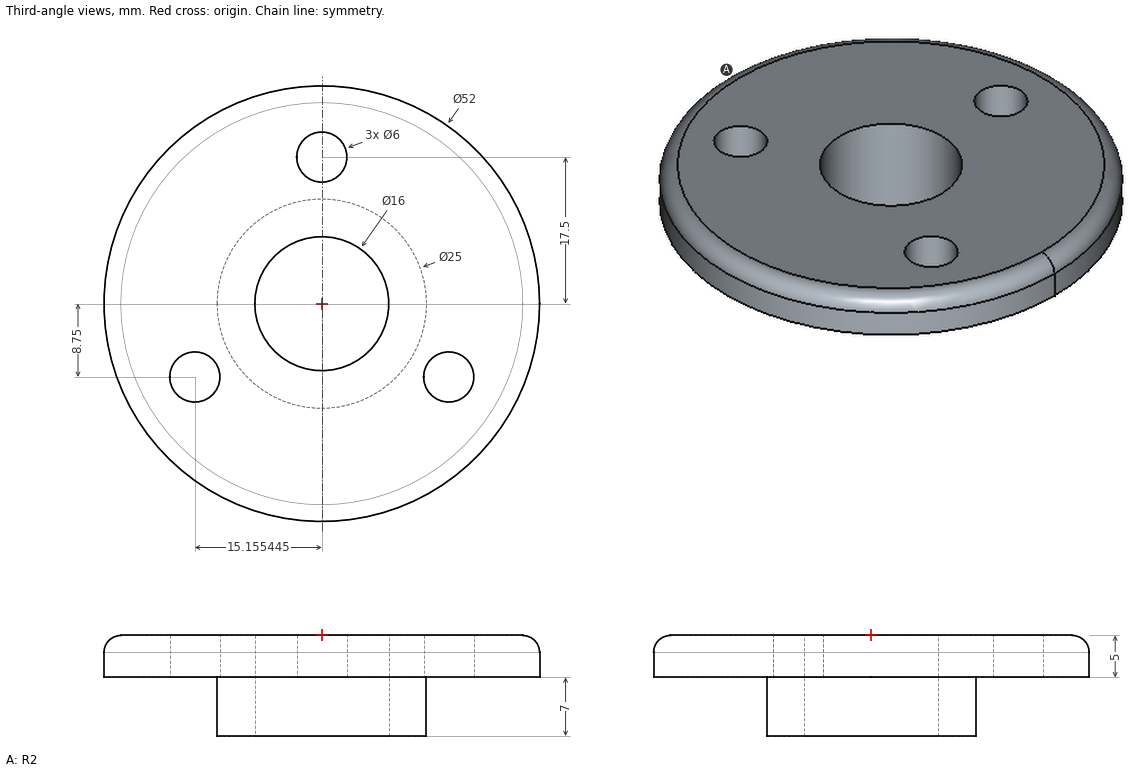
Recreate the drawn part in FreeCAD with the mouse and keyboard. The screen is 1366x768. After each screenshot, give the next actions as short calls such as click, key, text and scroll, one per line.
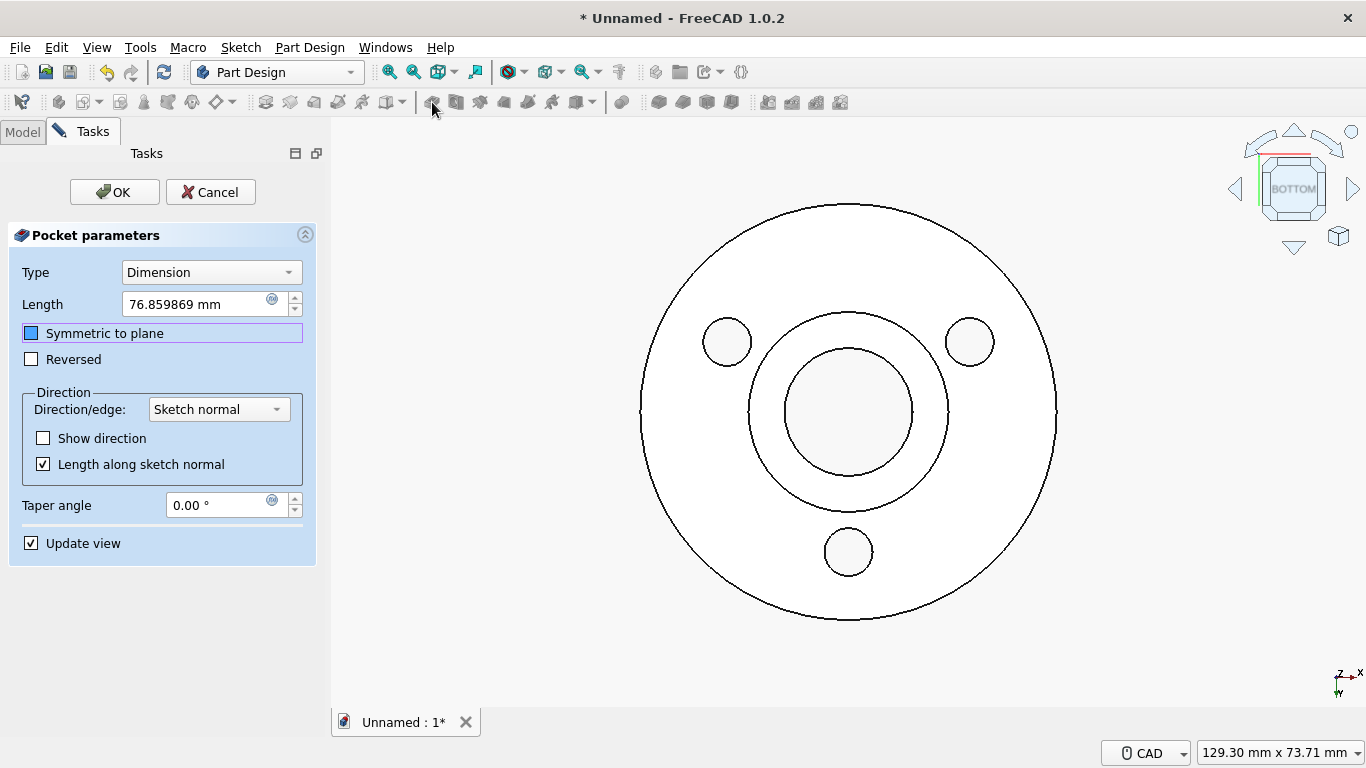
click(30, 333)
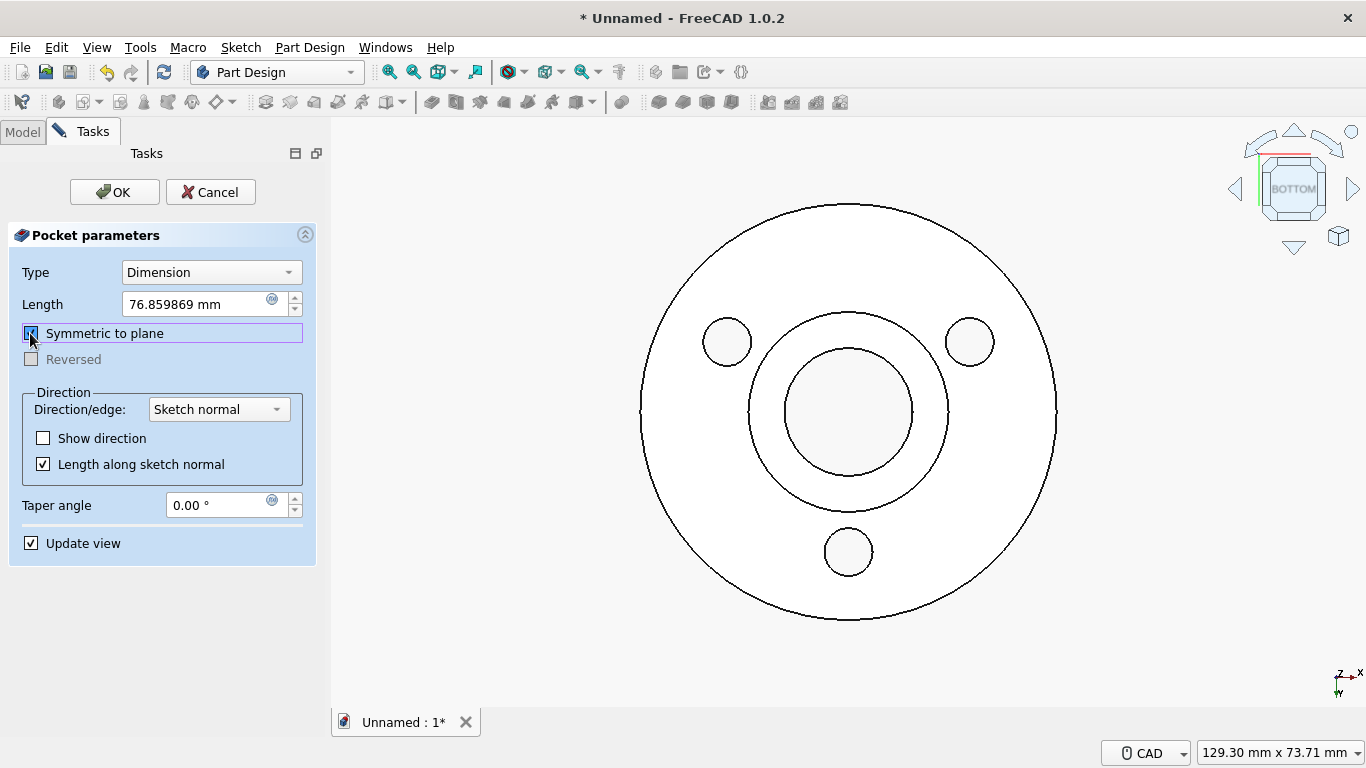
click(115, 192)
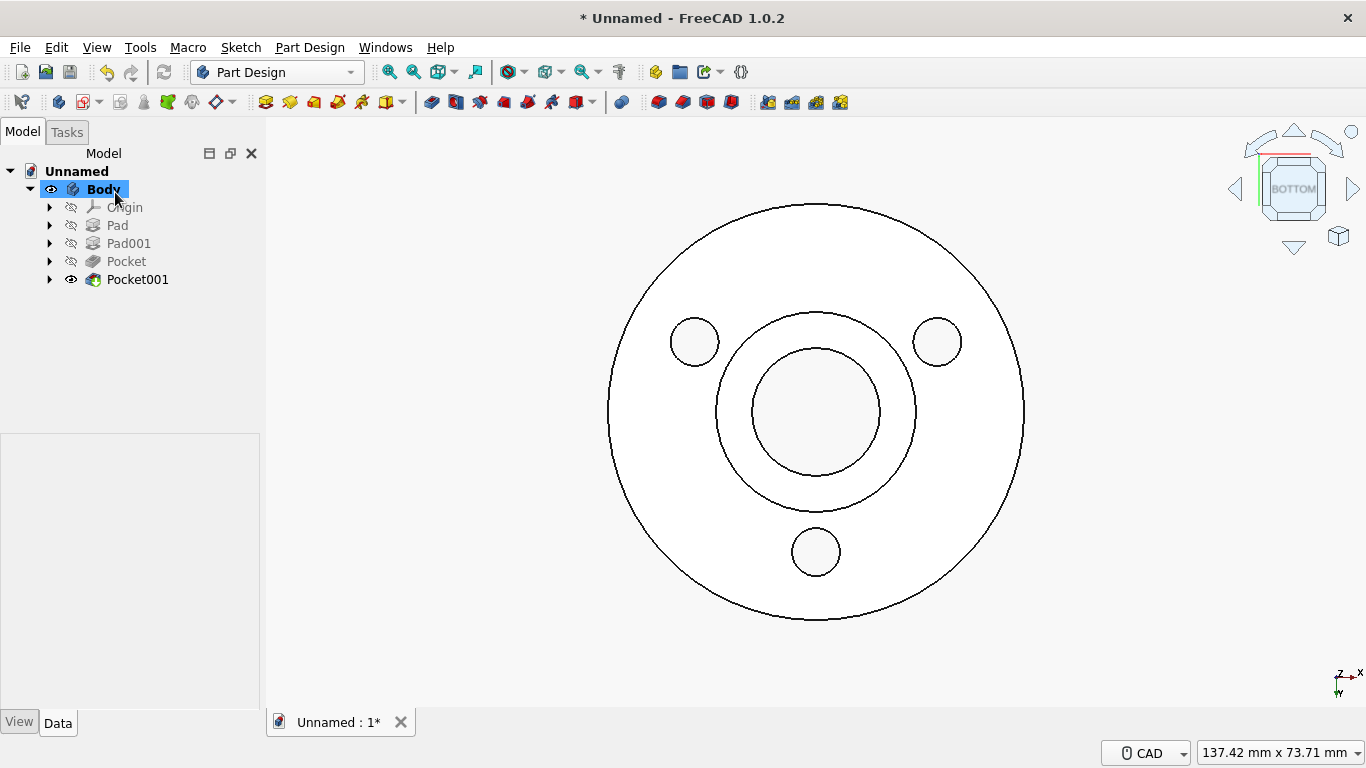
key(0)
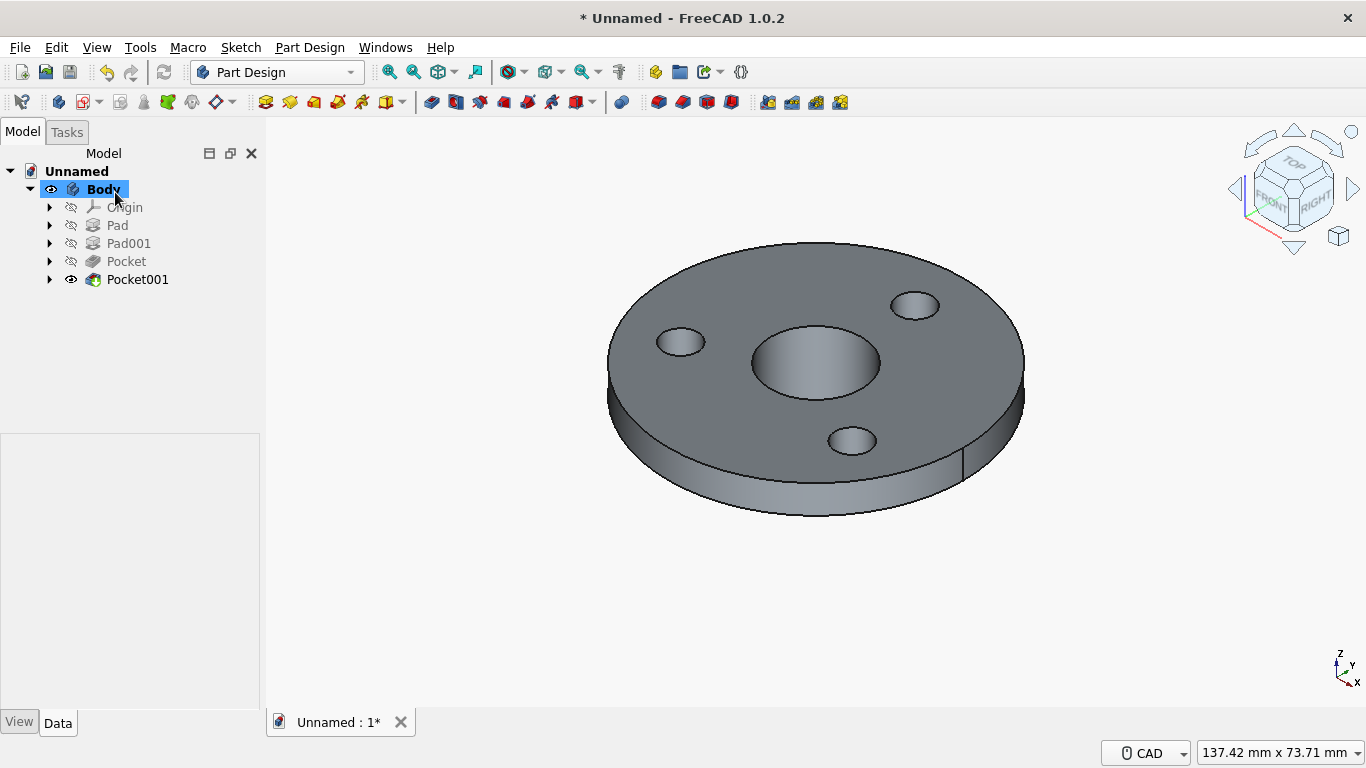
click(631, 417)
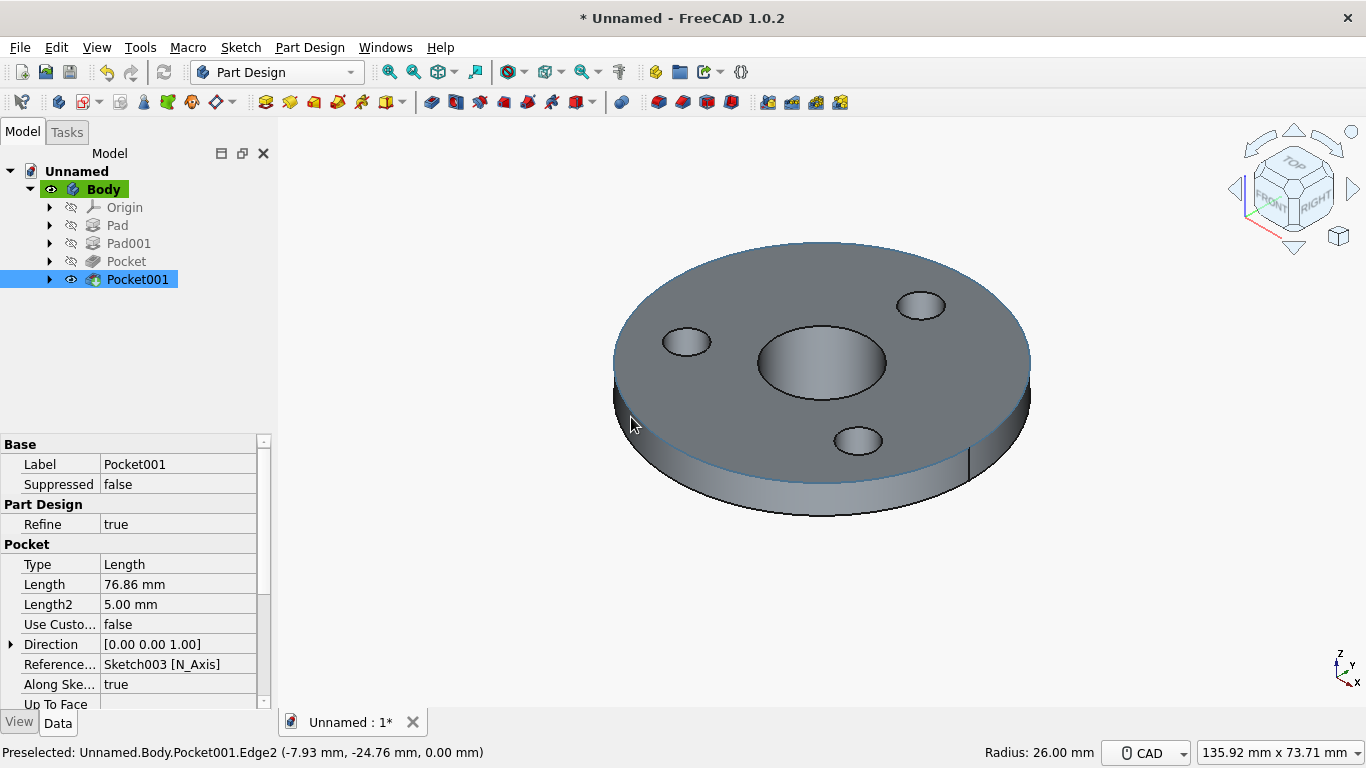
click(660, 102)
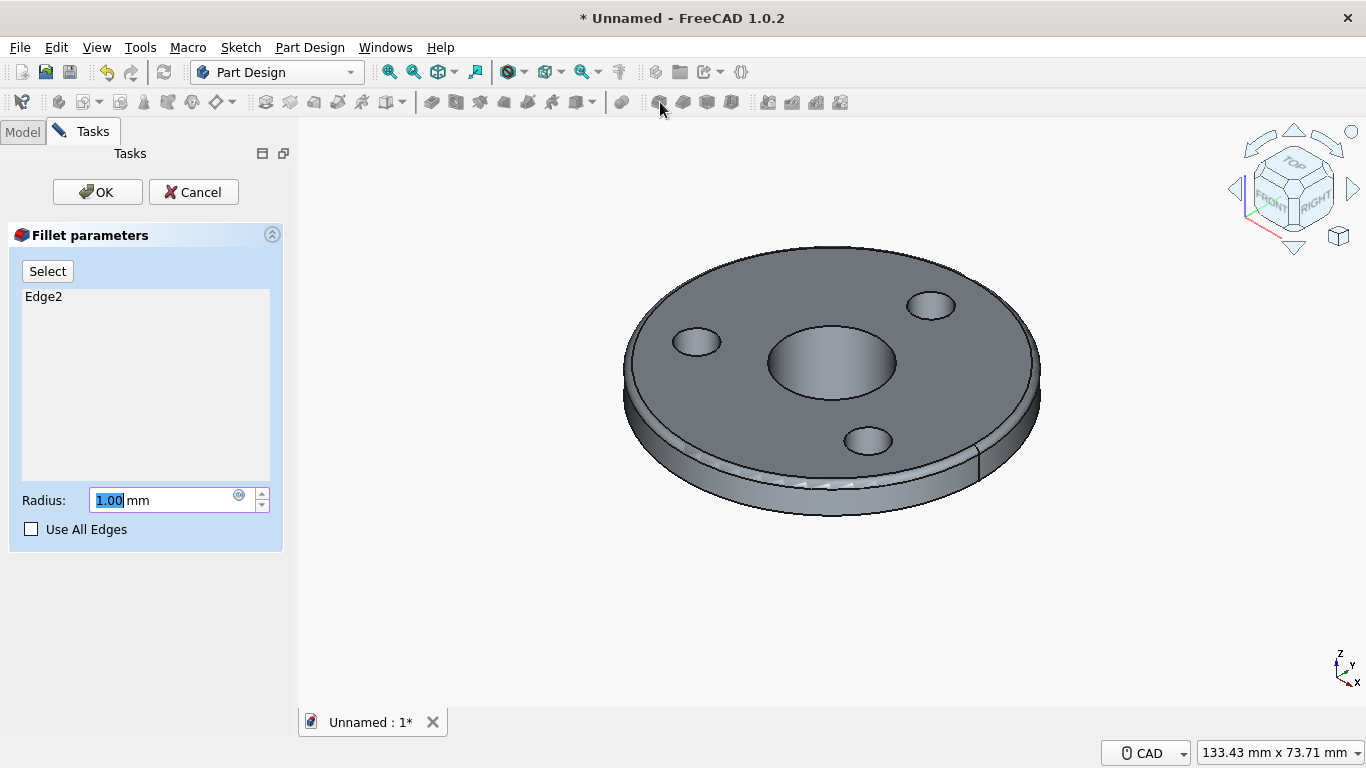
text(2)
key(Tab)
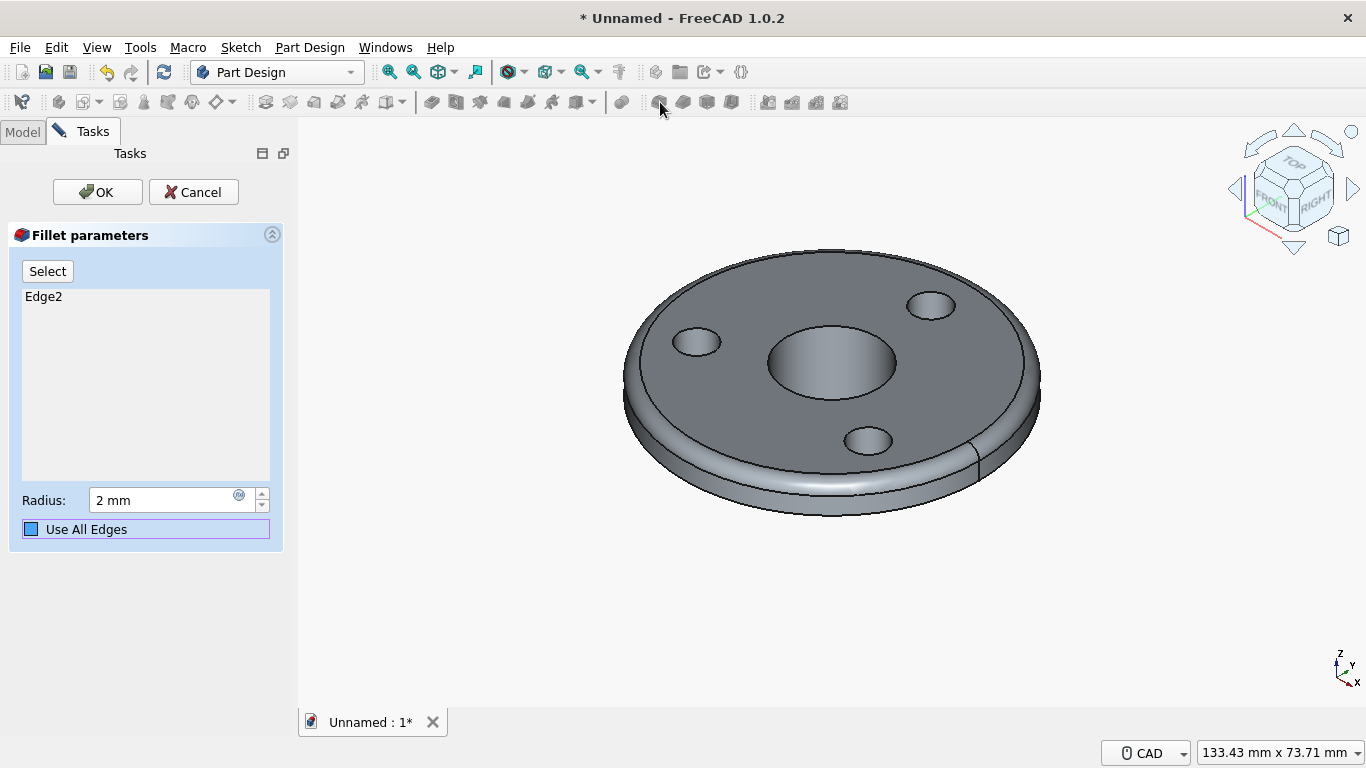
click(98, 192)